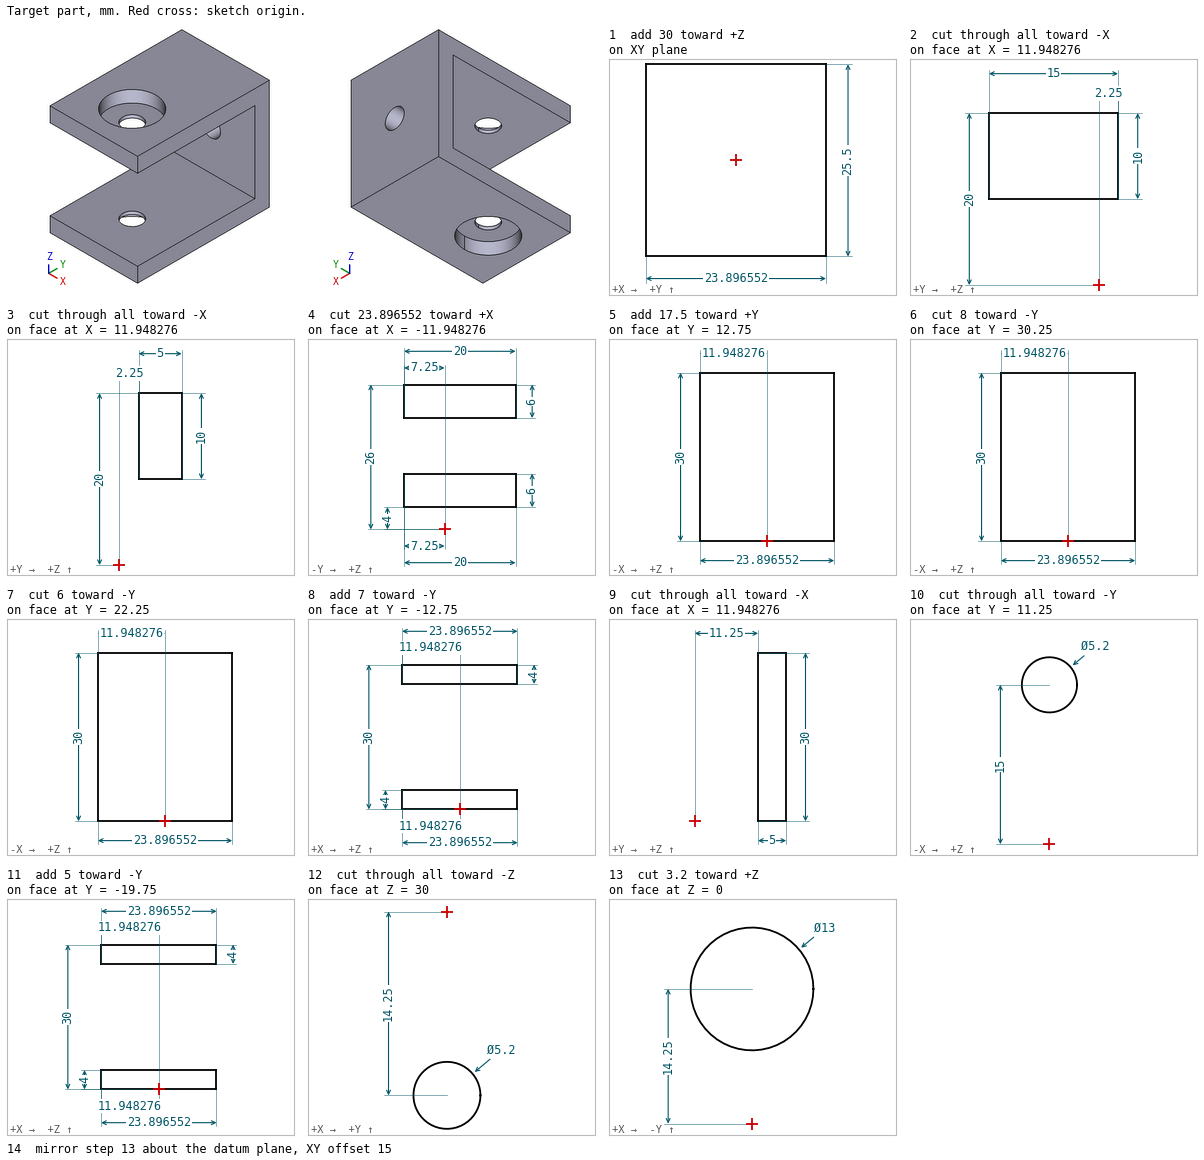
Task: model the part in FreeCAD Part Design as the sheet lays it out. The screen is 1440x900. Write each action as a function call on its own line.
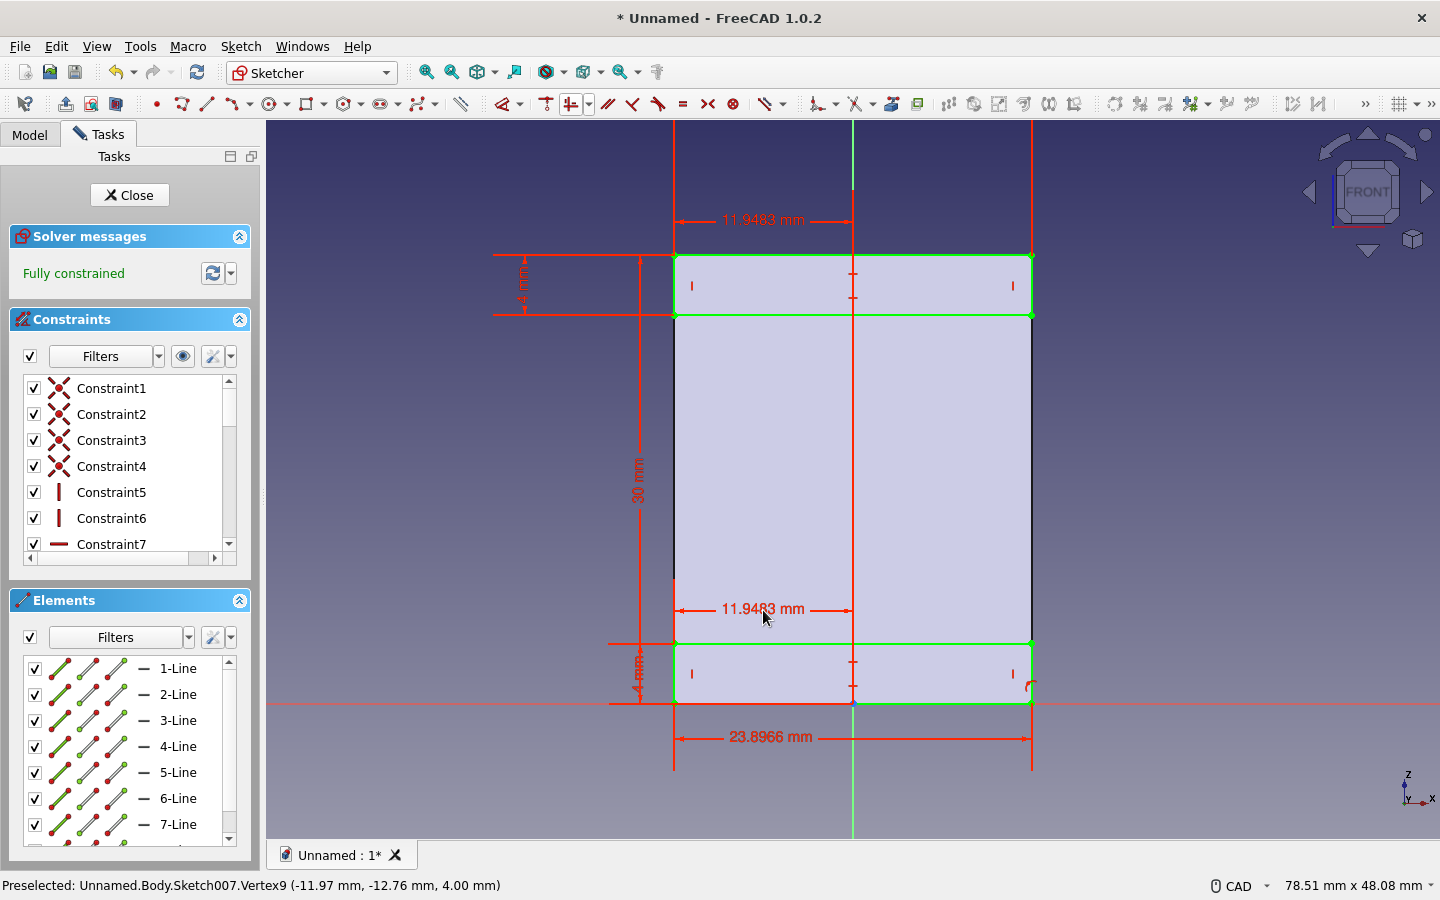
click(130, 195)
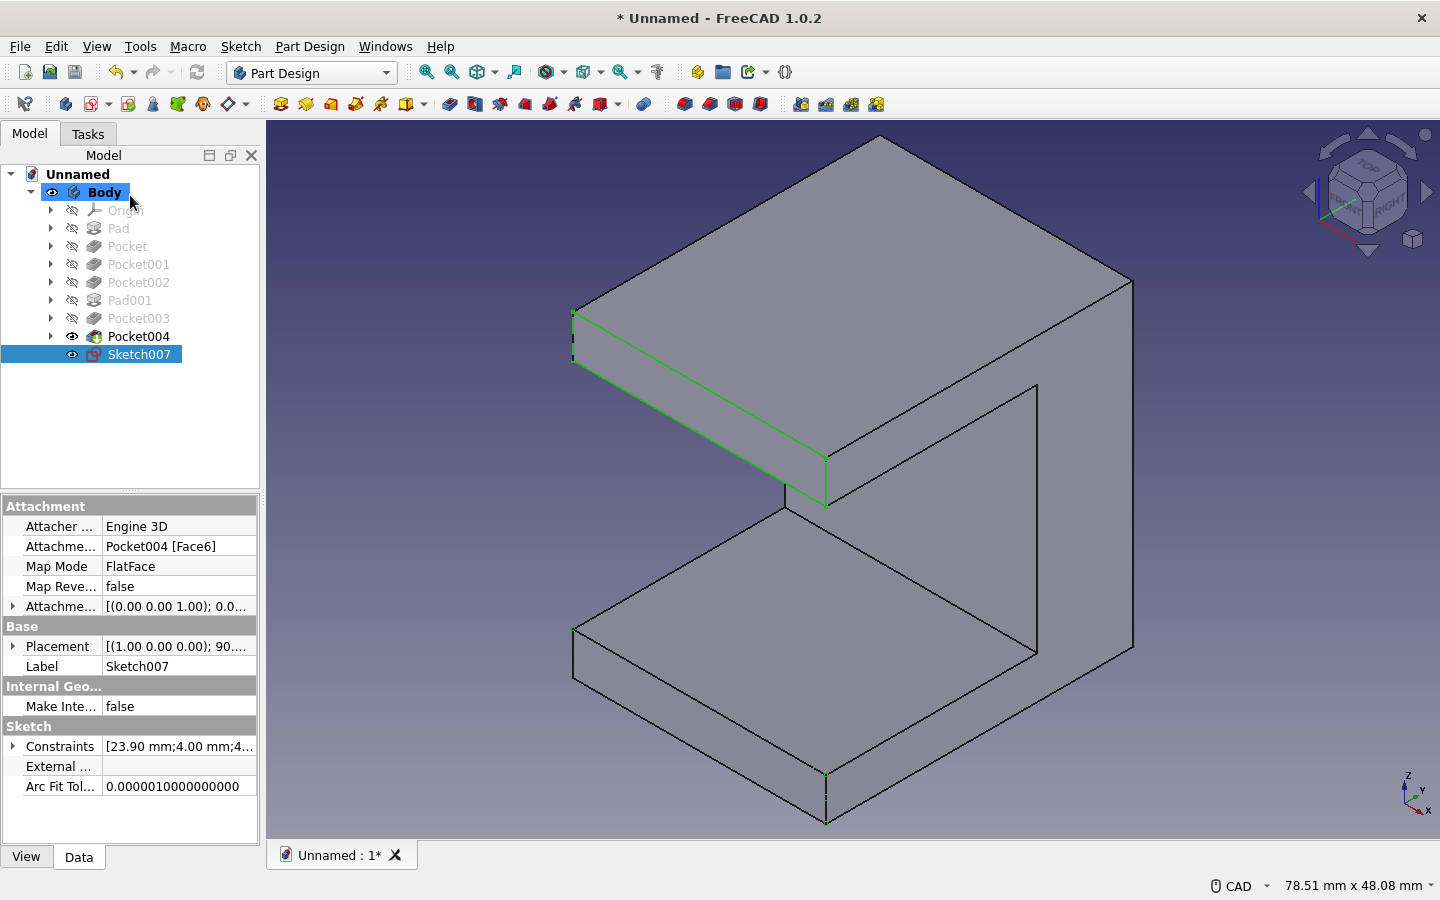
click(281, 104)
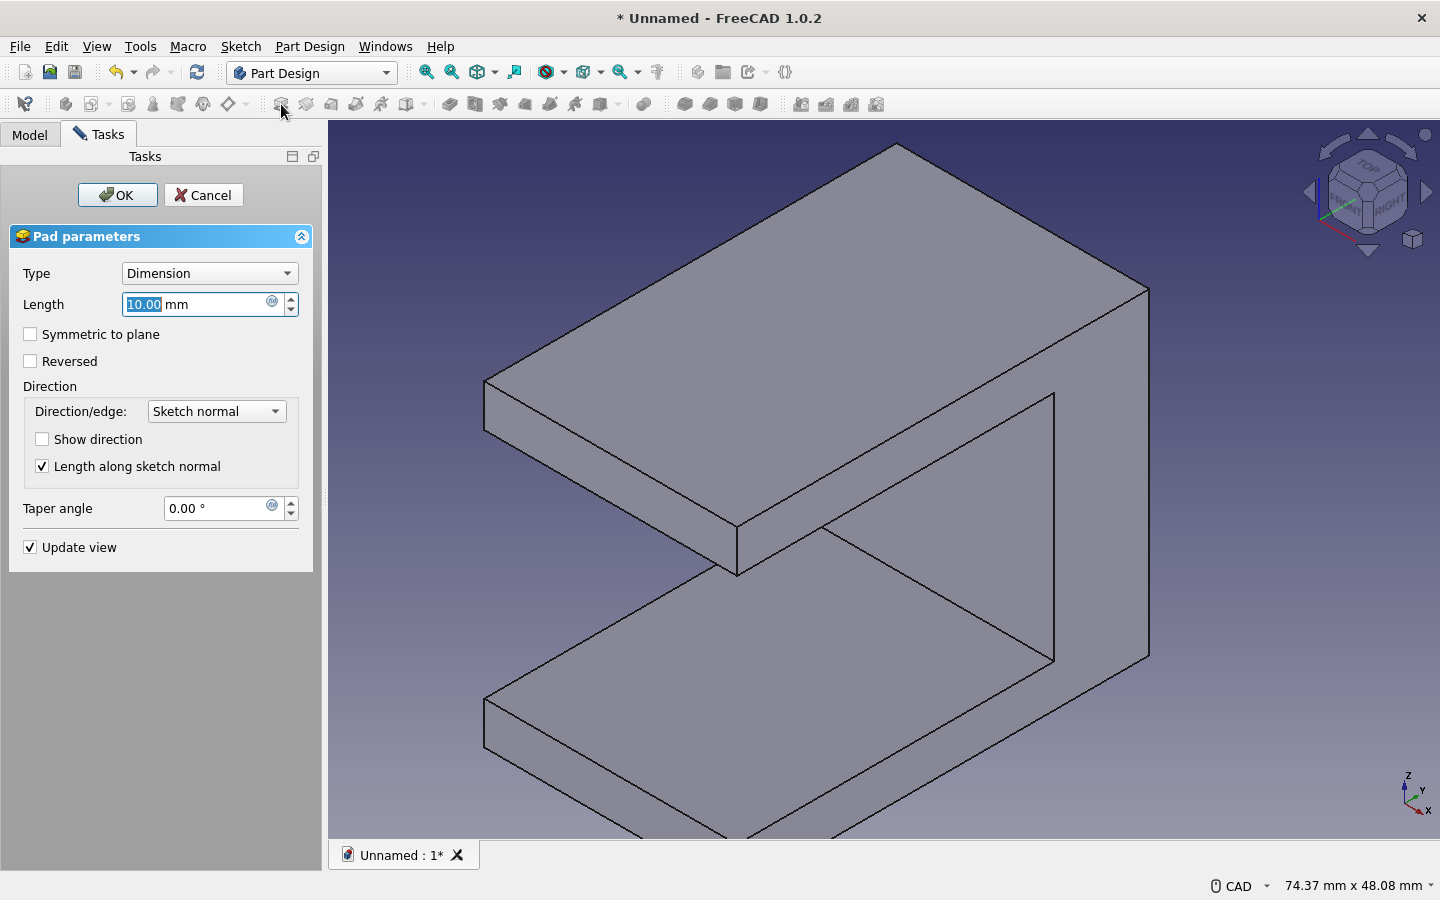
text(7)
key(Tab)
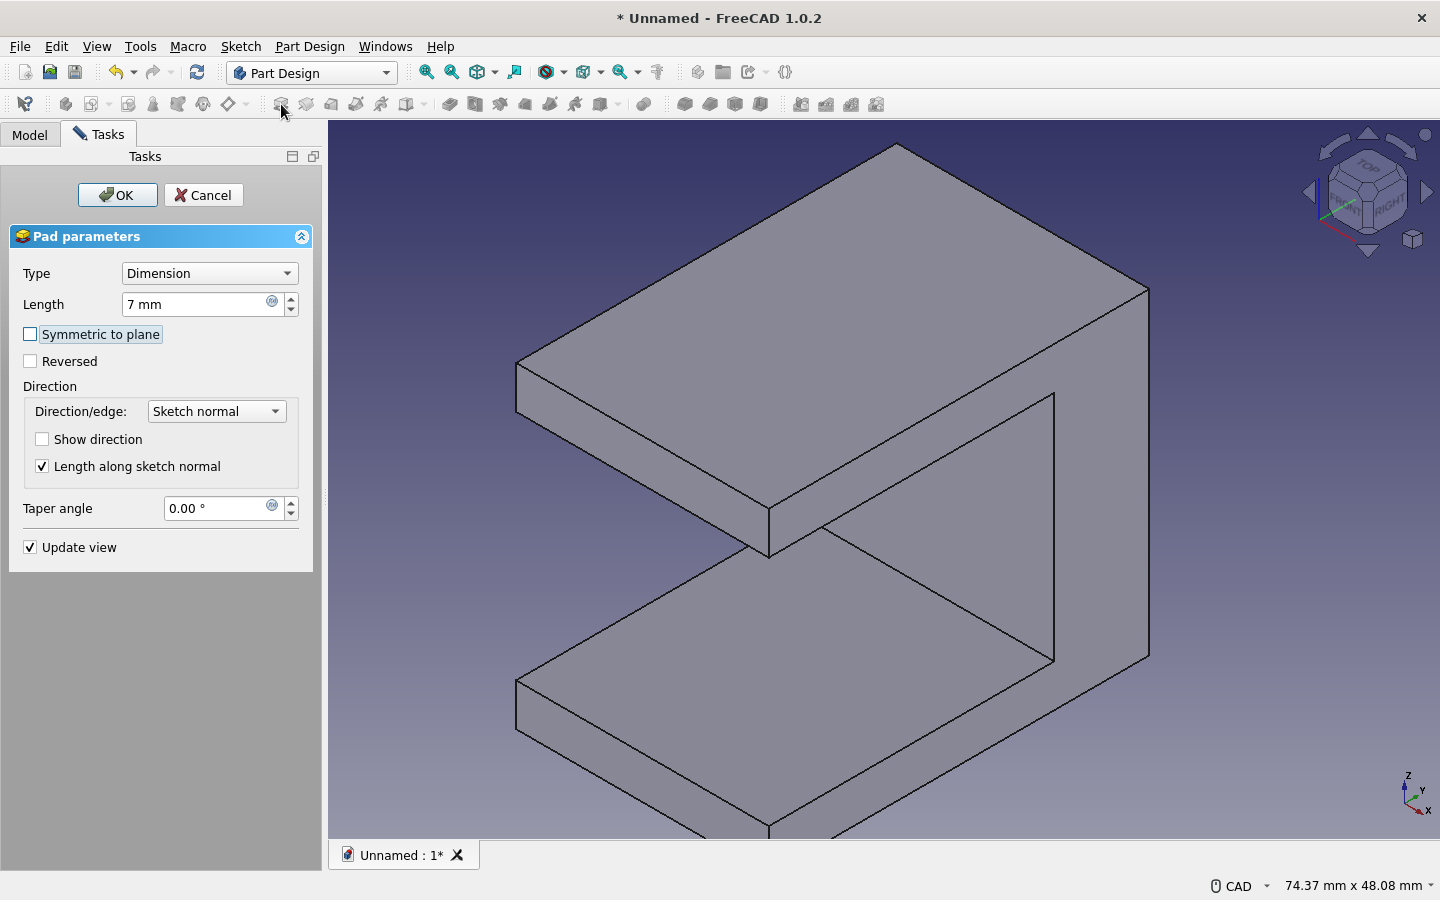
click(118, 195)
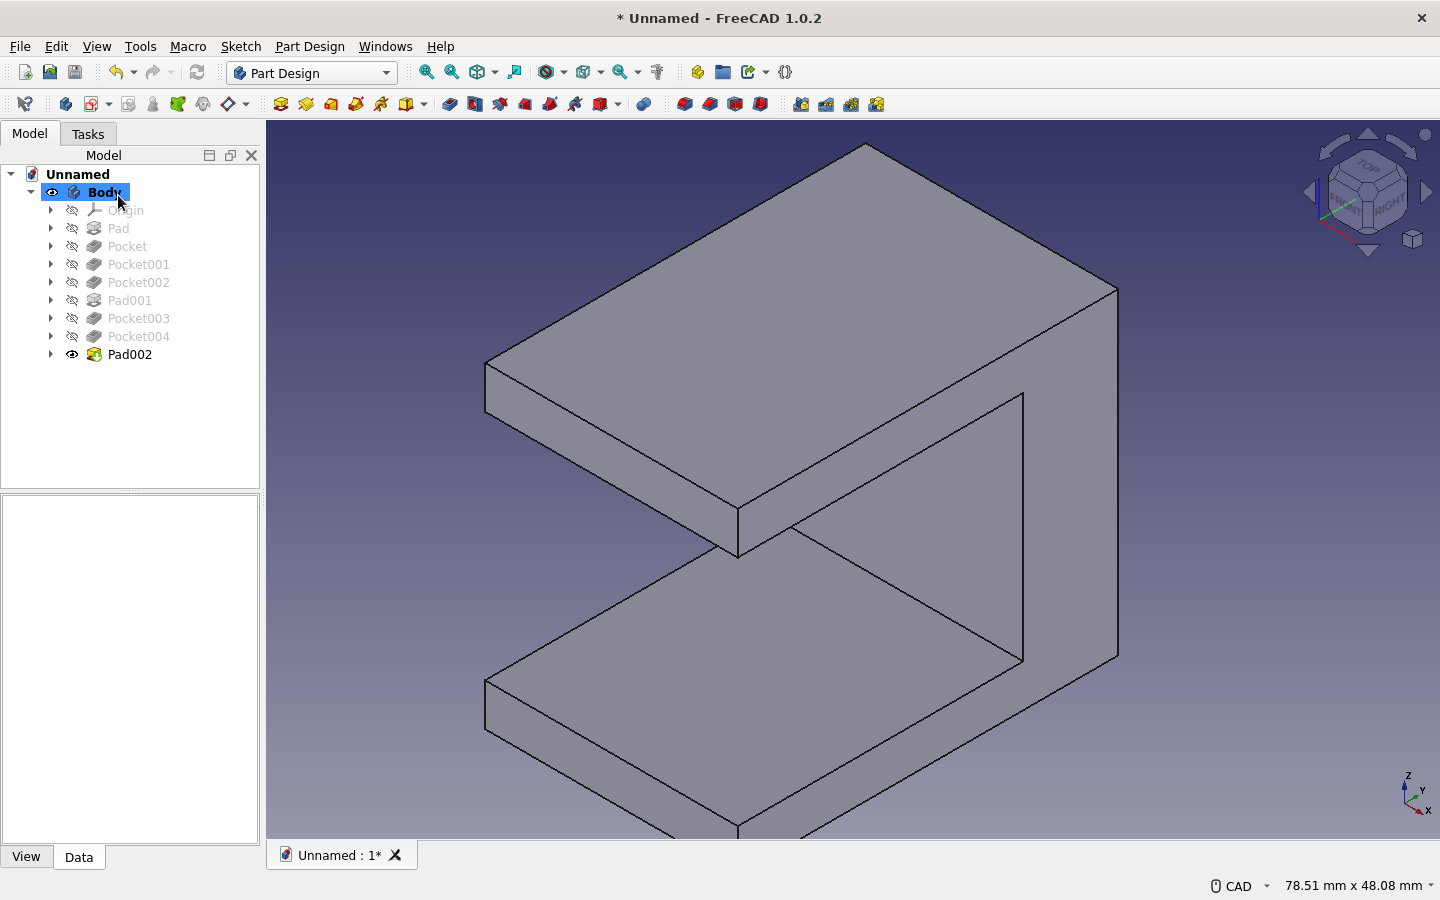
key(v)
key(f)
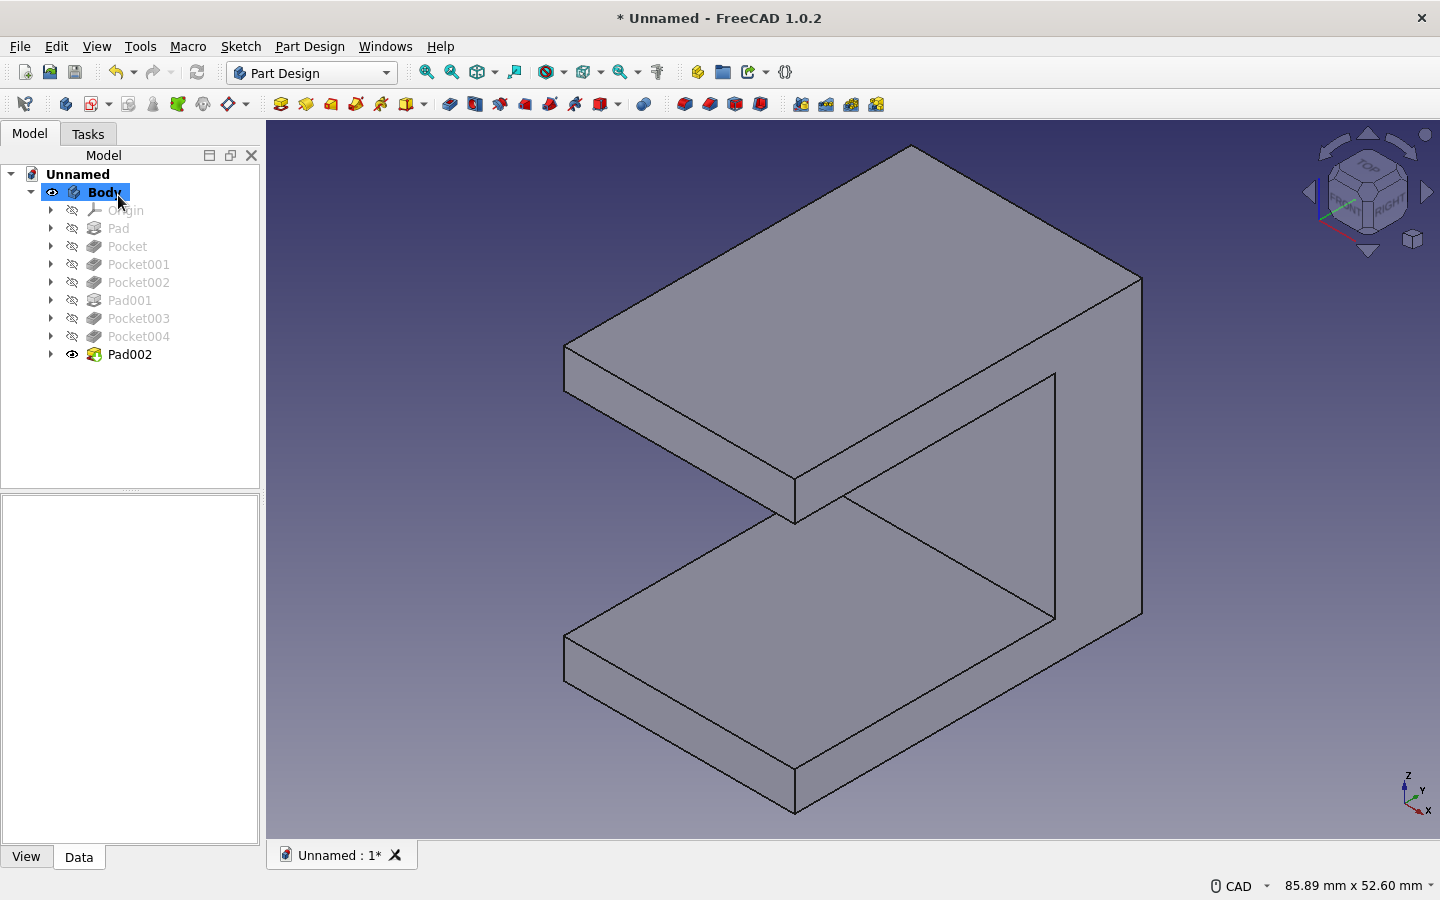
click(1118, 363)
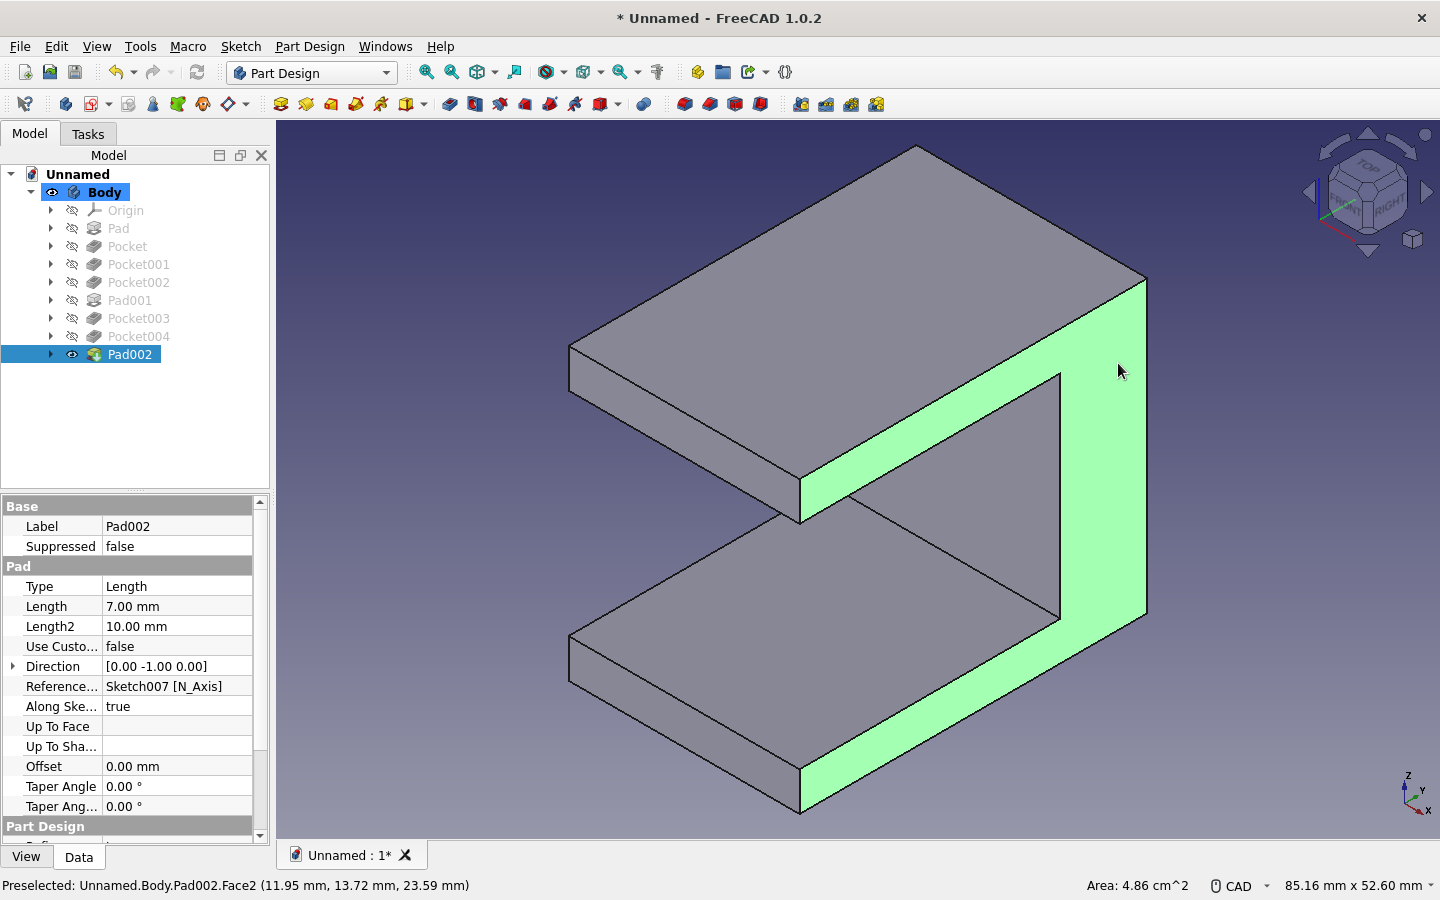
click(90, 104)